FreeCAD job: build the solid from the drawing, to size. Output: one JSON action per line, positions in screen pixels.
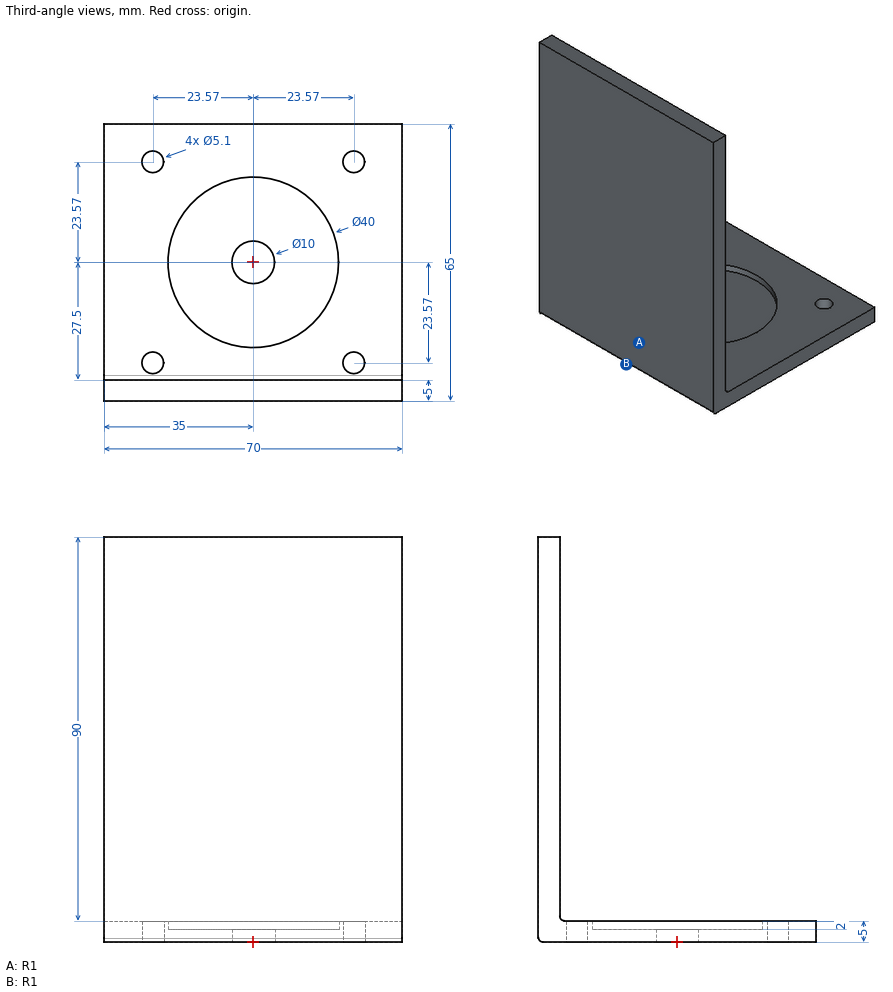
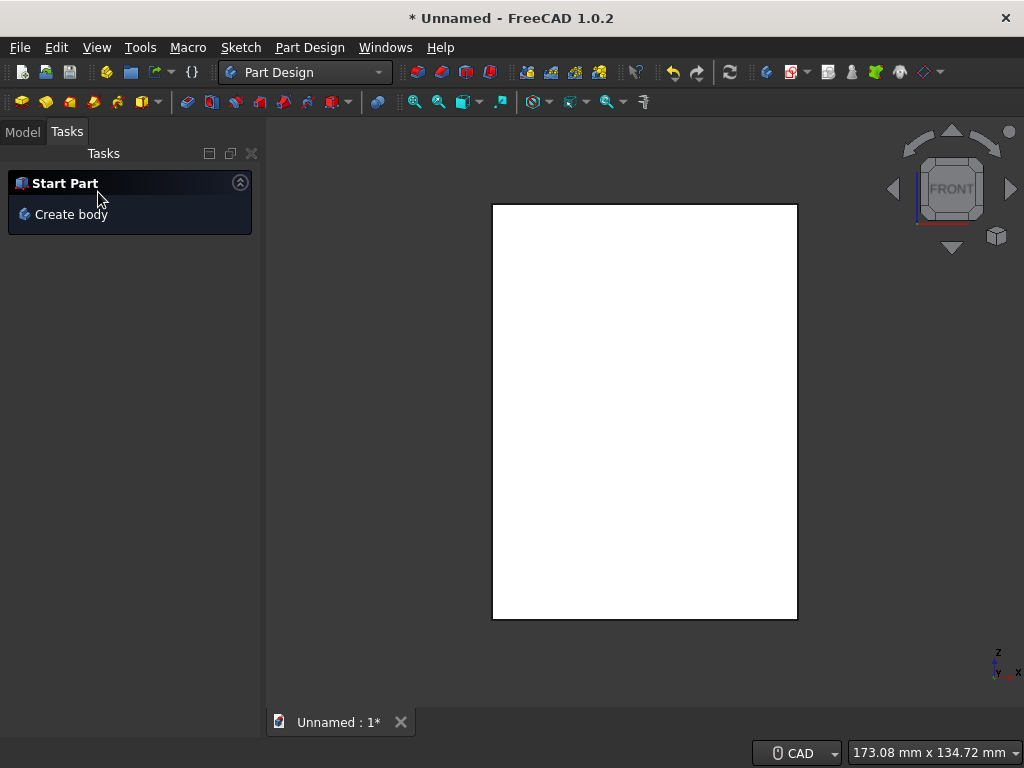
{"action": "left_click", "coordinate": [645, 619]}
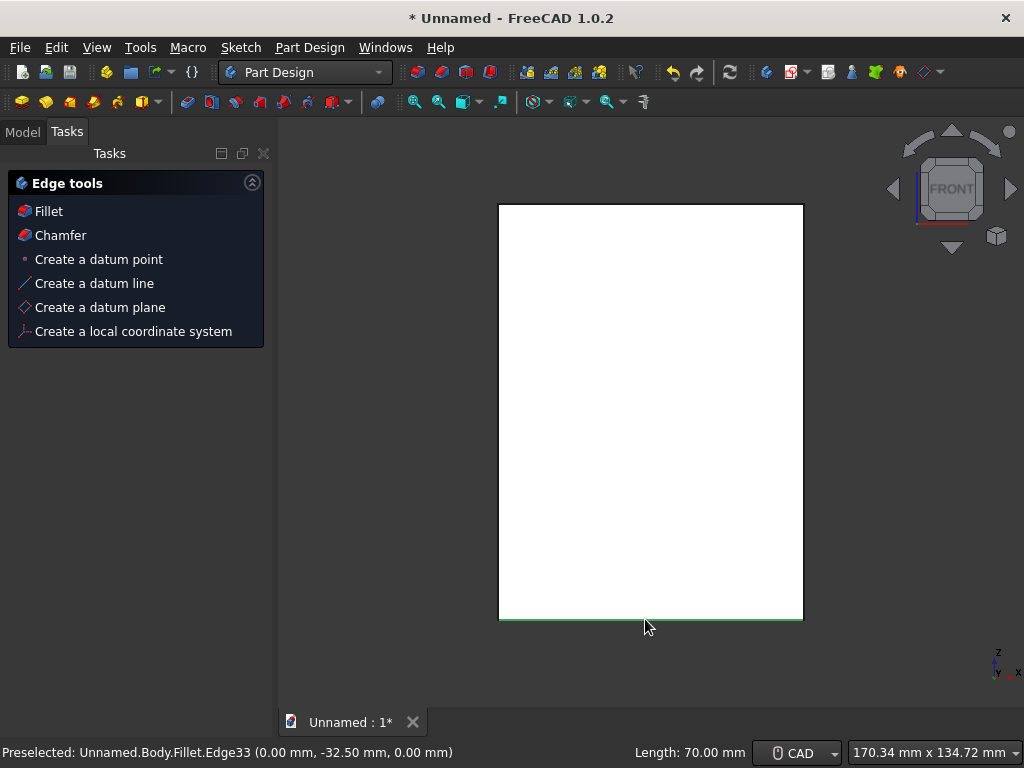
{"action": "left_click", "coordinate": [418, 72]}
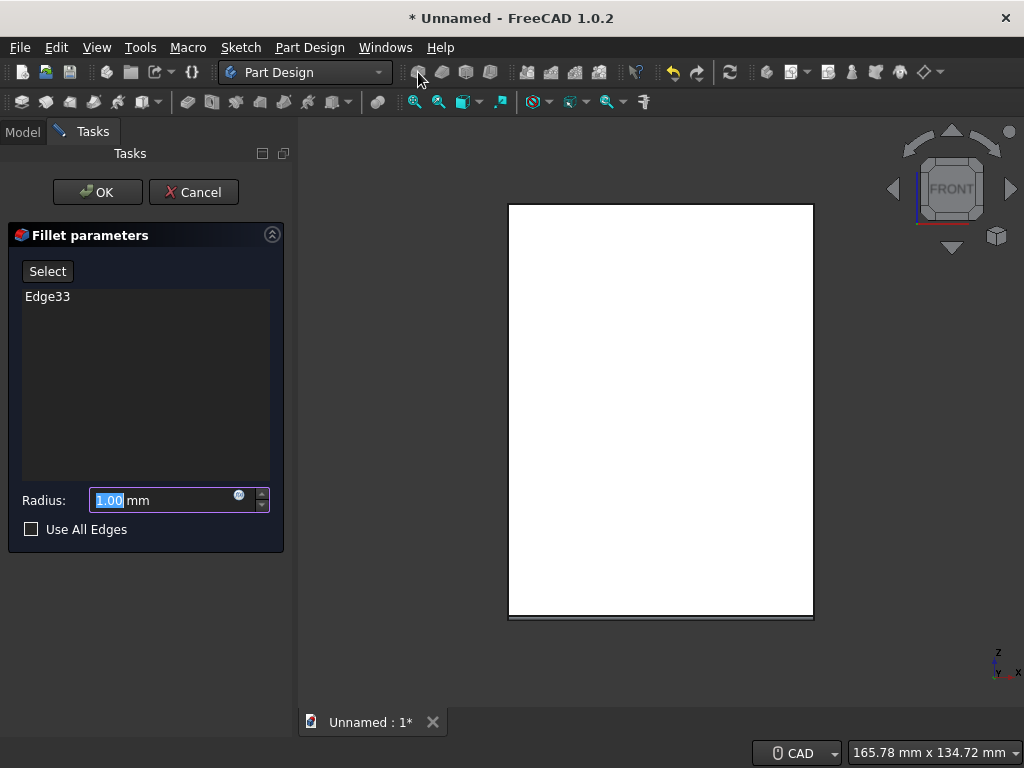
{"action": "type", "text": "1"}
{"action": "key", "text": "Tab"}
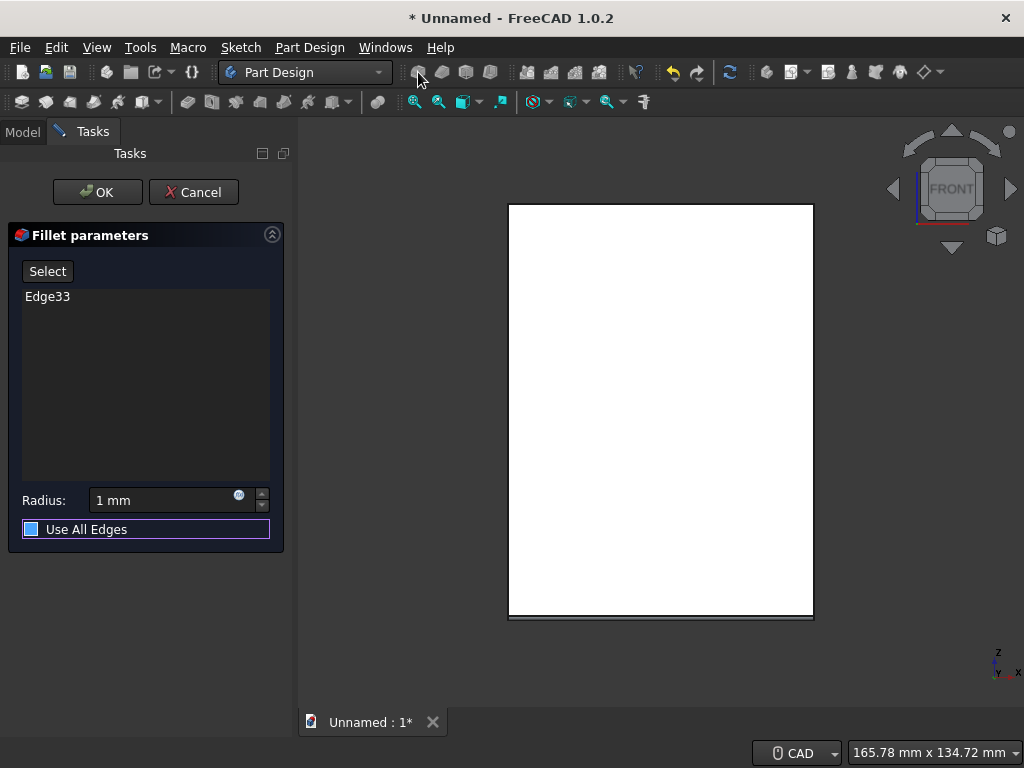
{"action": "left_click", "coordinate": [98, 192]}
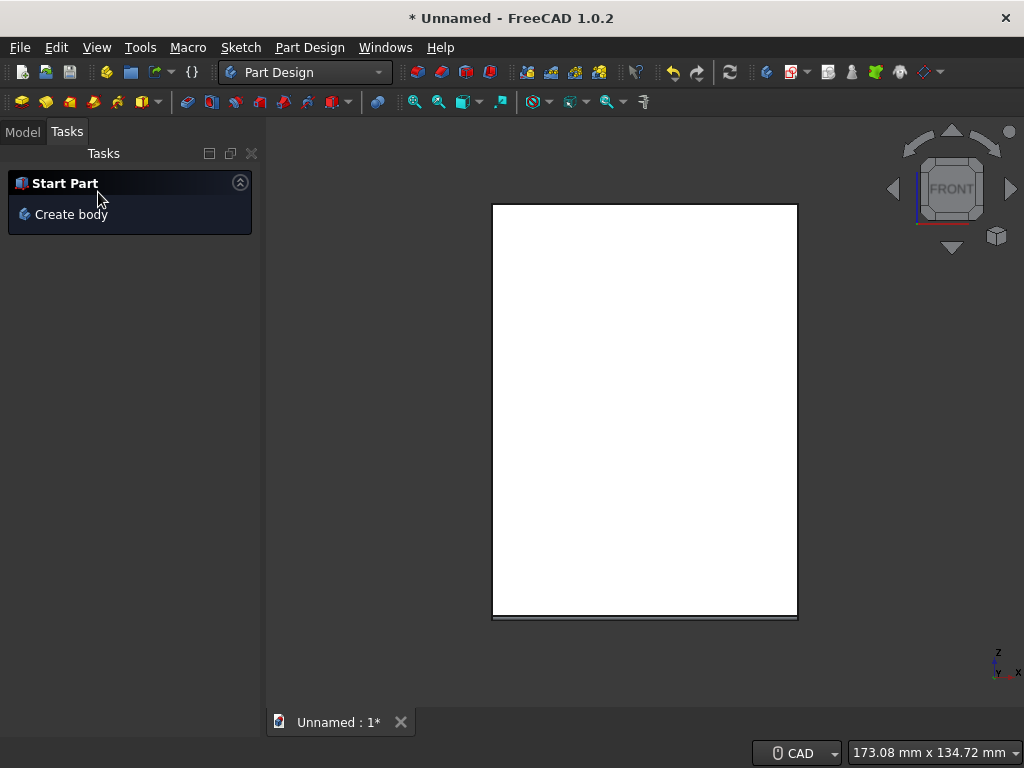
{"action": "key", "text": "0"}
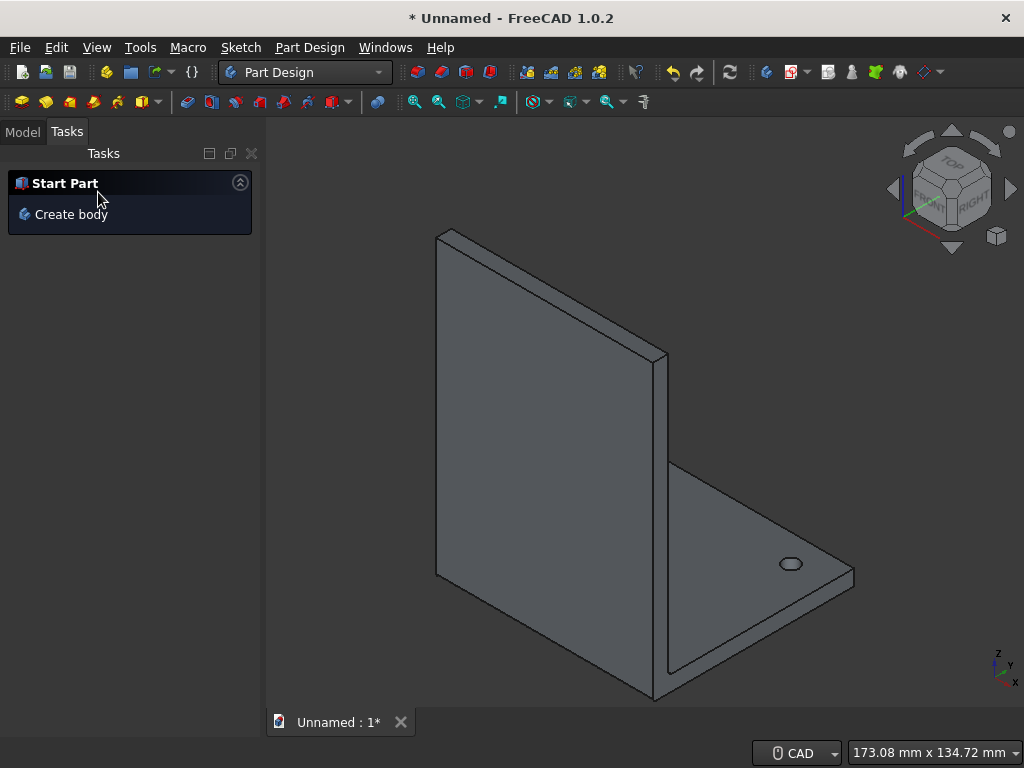
{"action": "left_click", "coordinate": [685, 575]}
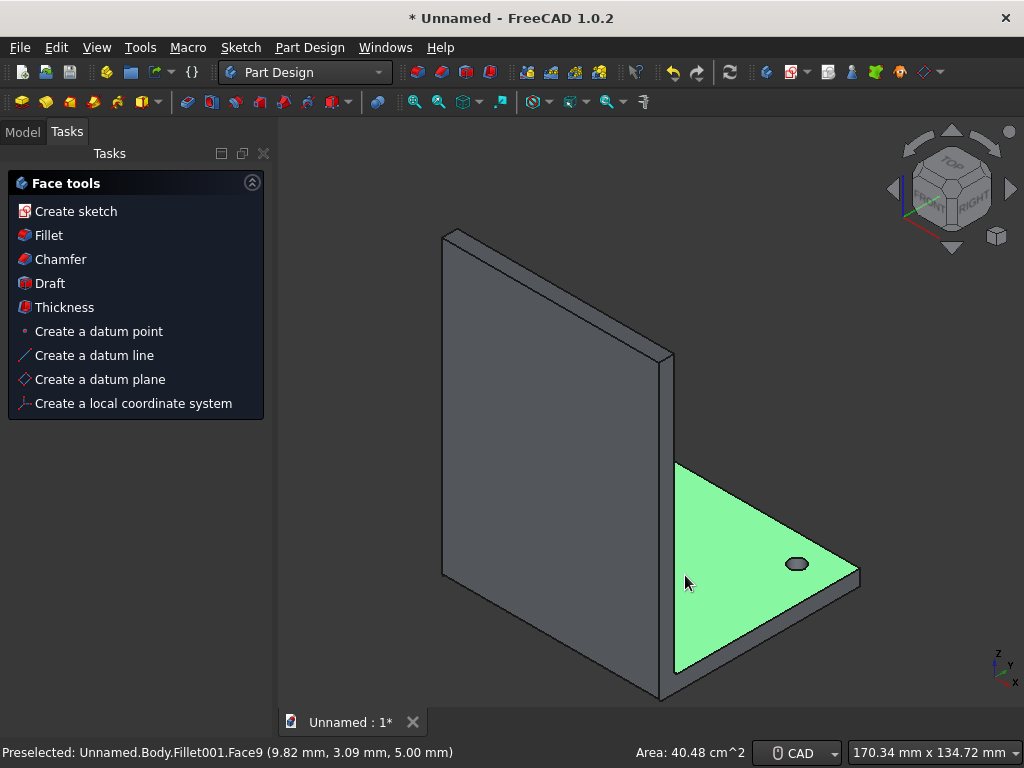
{"action": "left_click", "coordinate": [792, 72]}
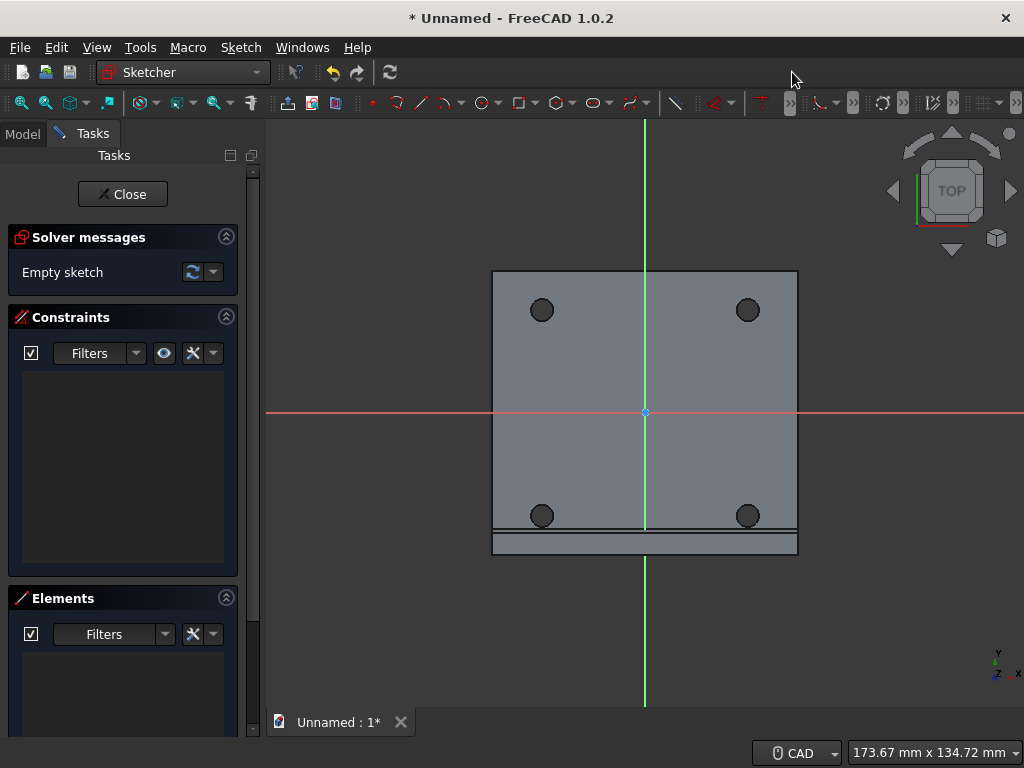
{"action": "scroll", "coordinate": [701, 413], "scroll_direction": "up", "scroll_amount": 4}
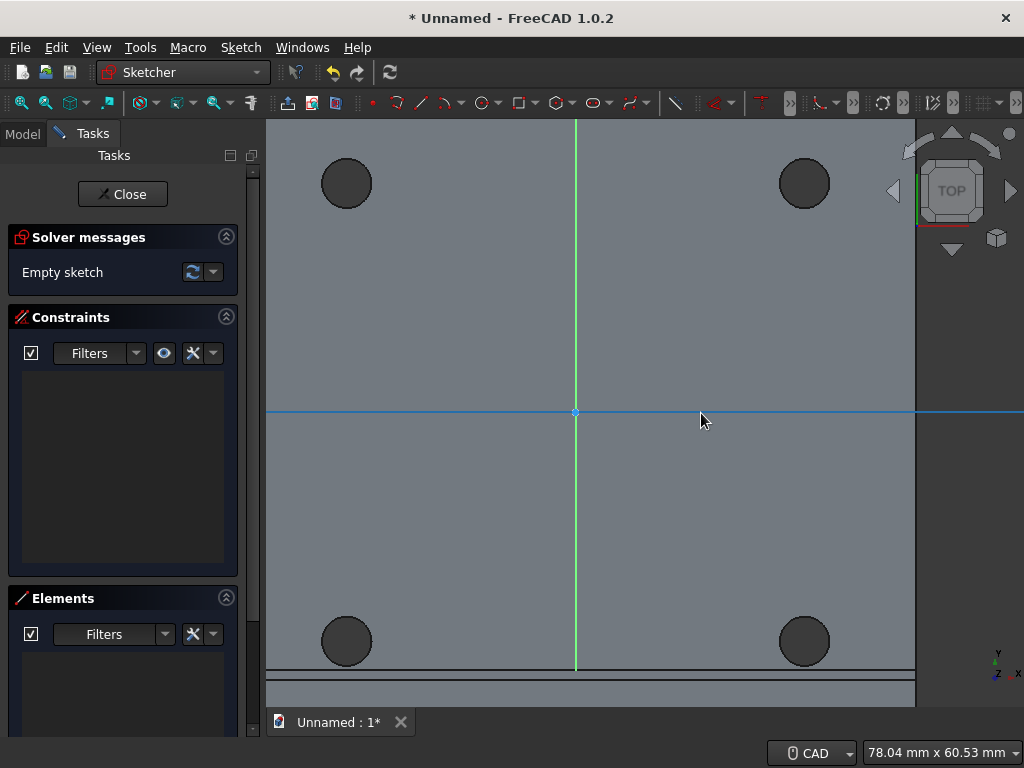
{"action": "left_click", "coordinate": [482, 104]}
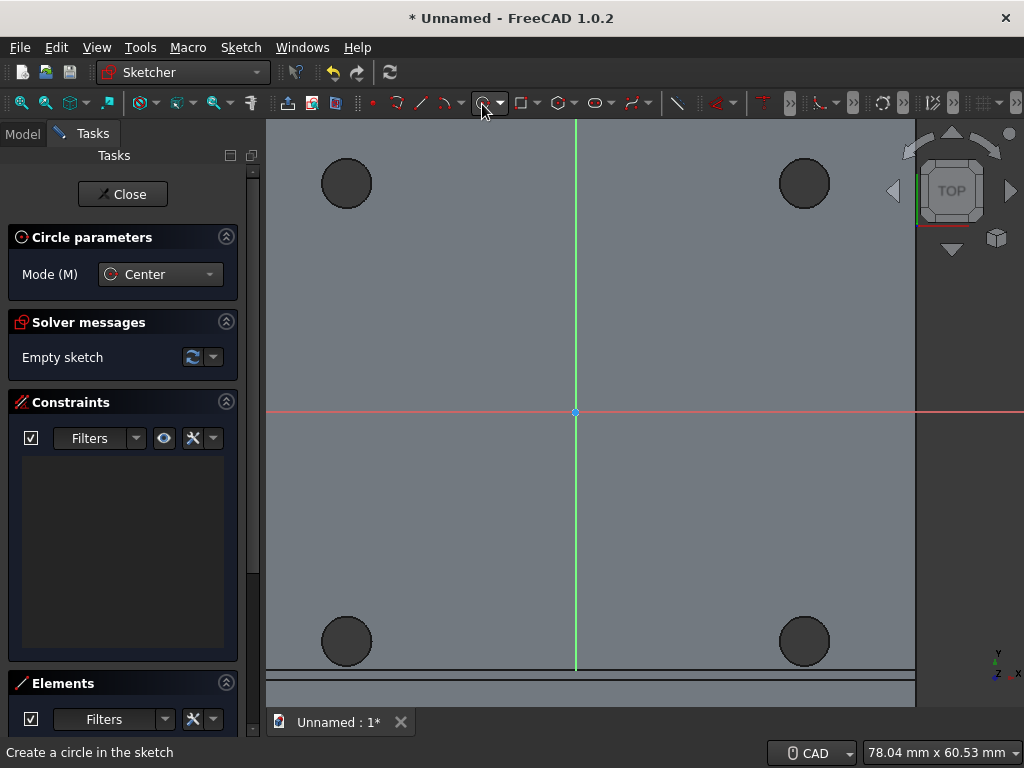
{"action": "left_click", "coordinate": [576, 412]}
{"action": "mouse_move", "coordinate": [713, 275]}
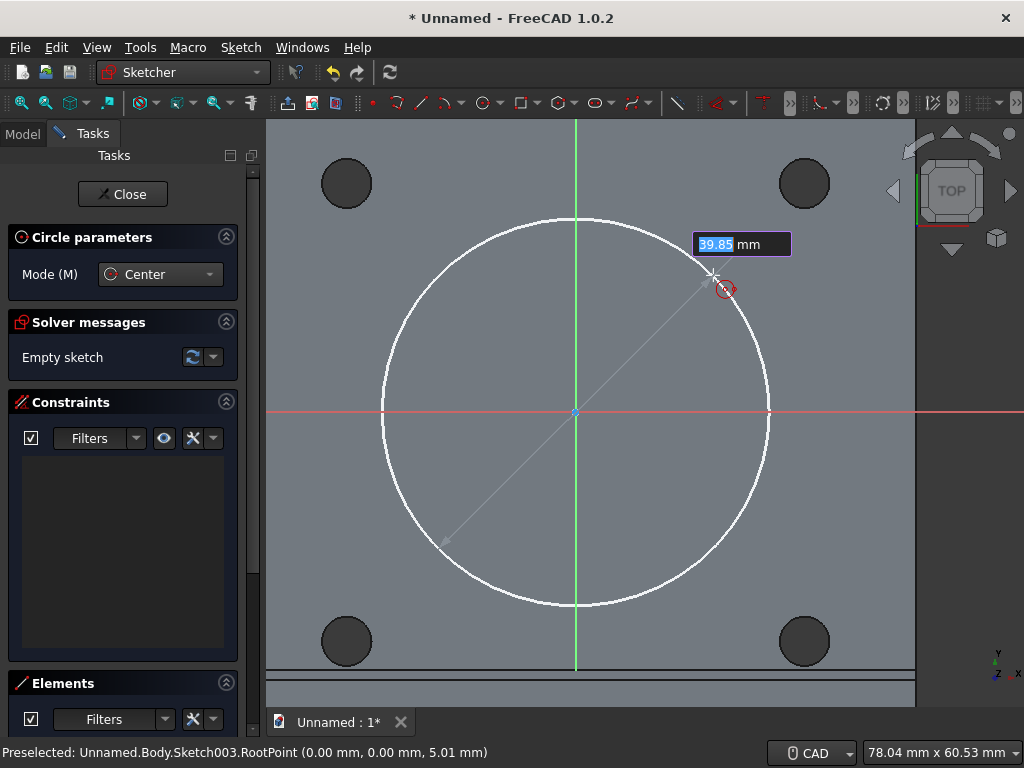
{"action": "type", "text": "40"}
{"action": "key", "text": "Return"}
{"action": "key", "text": "Escape"}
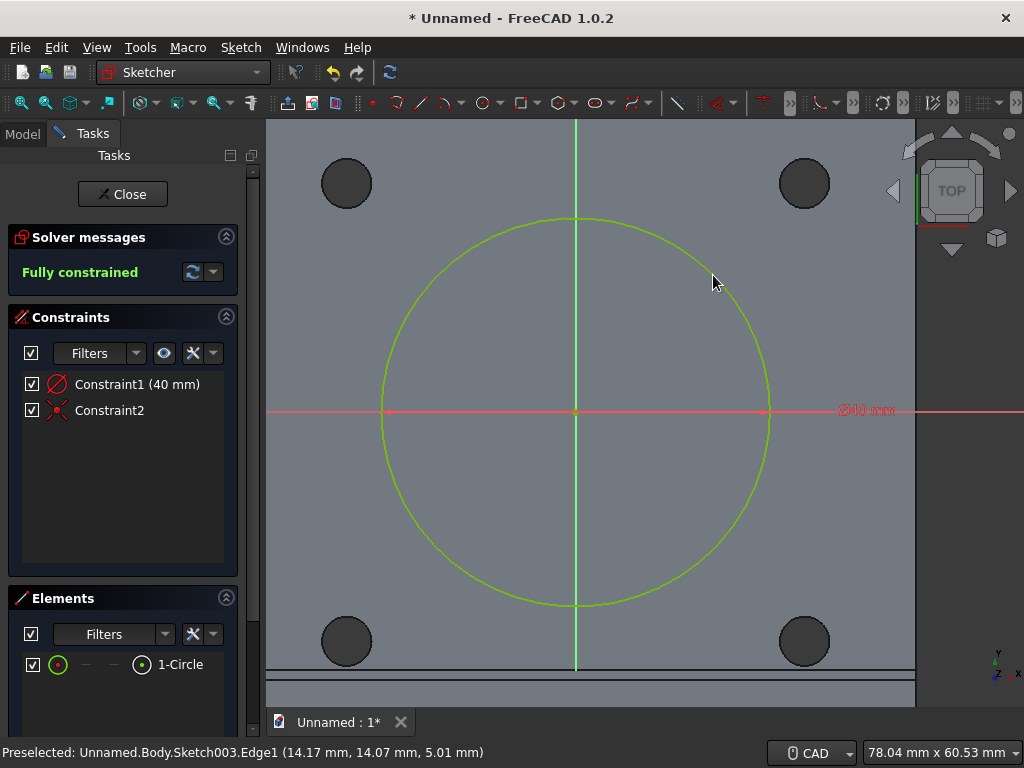
{"action": "left_click", "coordinate": [123, 194]}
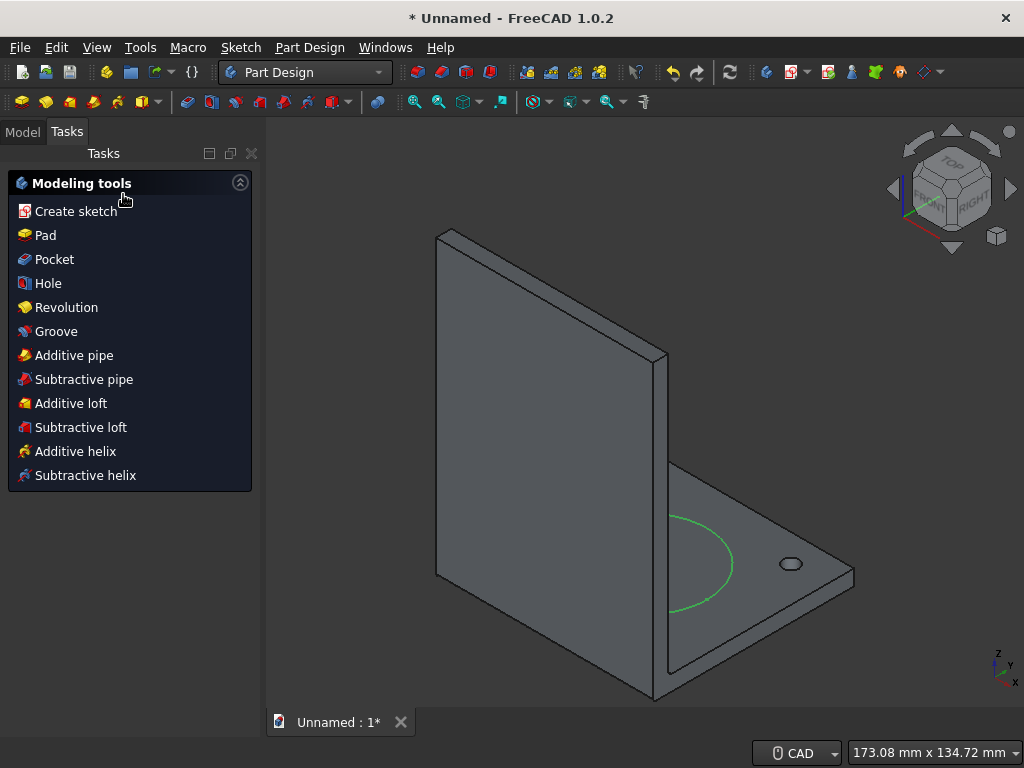
{"action": "left_click", "coordinate": [188, 102]}